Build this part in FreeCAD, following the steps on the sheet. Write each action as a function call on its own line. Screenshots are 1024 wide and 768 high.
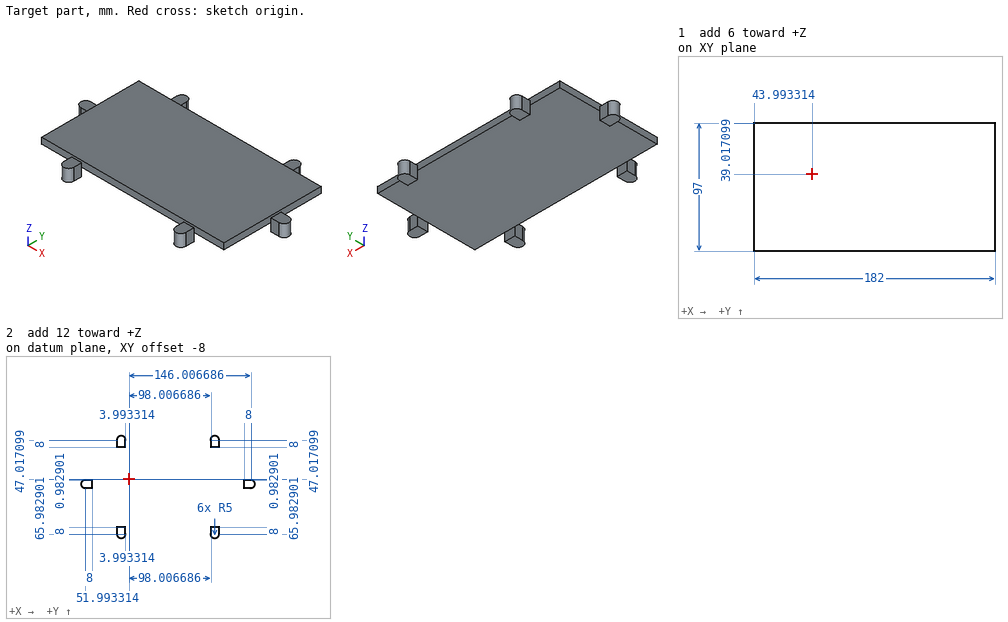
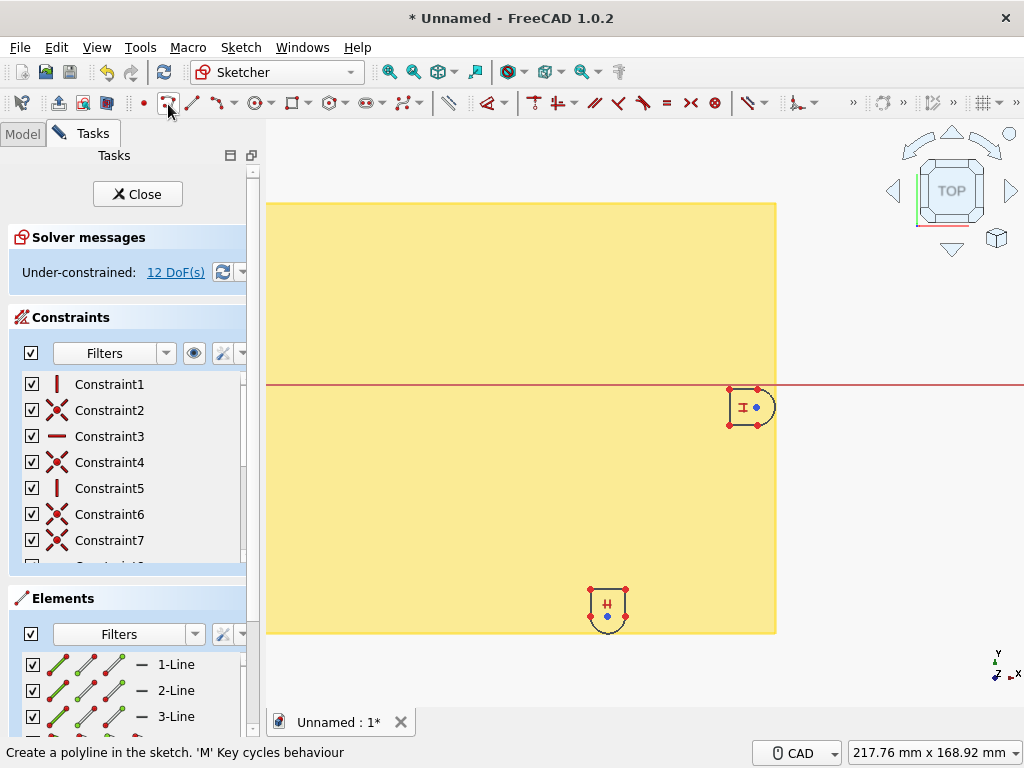
click(590, 222)
click(590, 250)
click(625, 250)
click(625, 222)
right_click(625, 222)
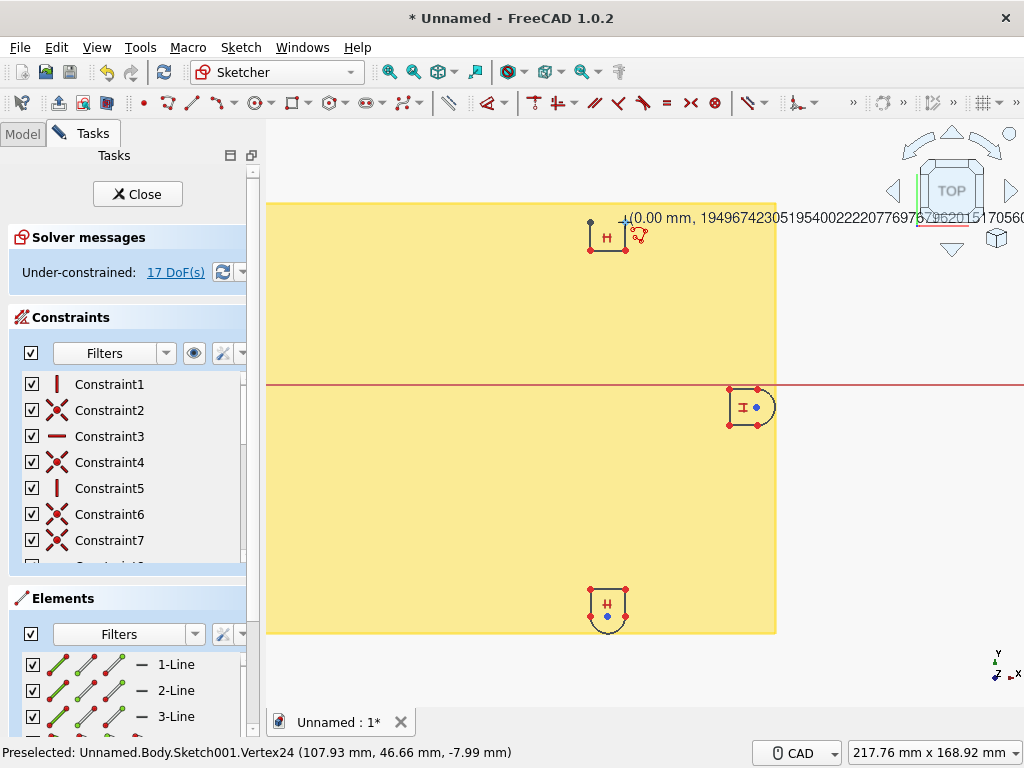
click(218, 104)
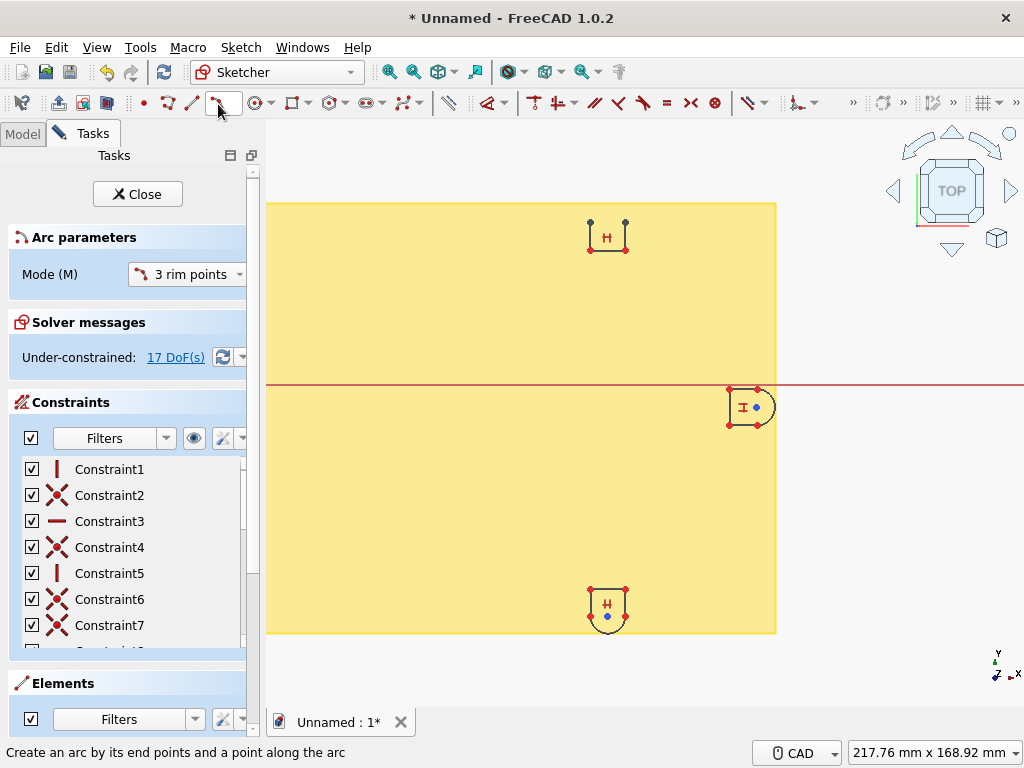
click(625, 223)
click(590, 223)
click(608, 204)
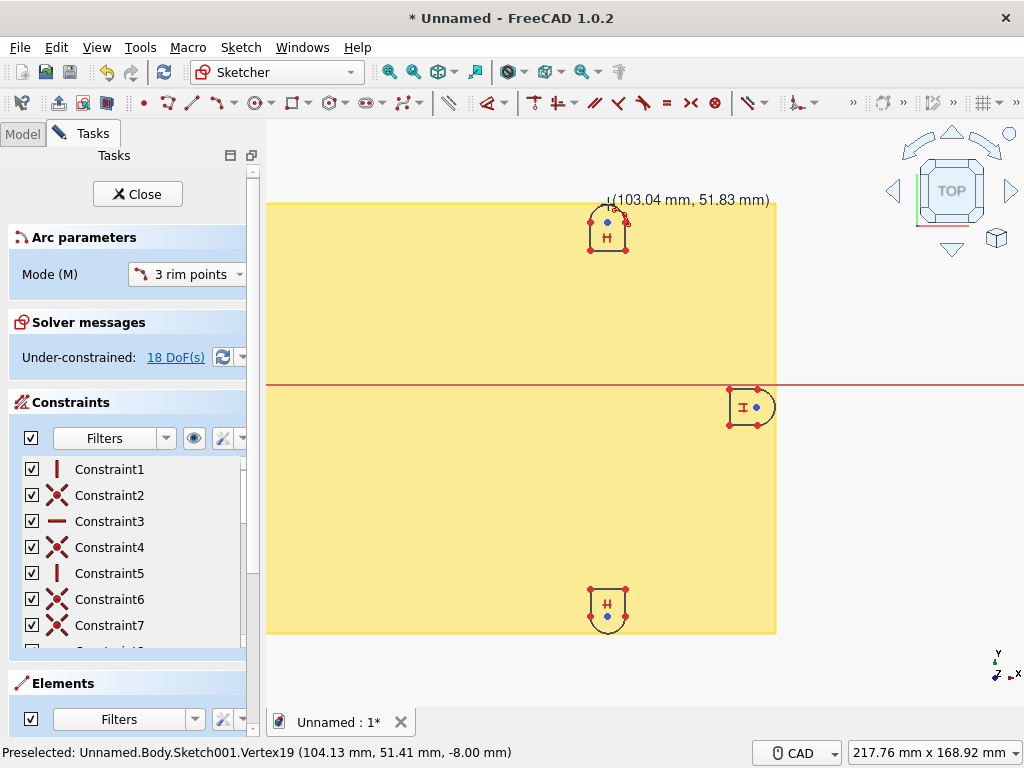
click(168, 104)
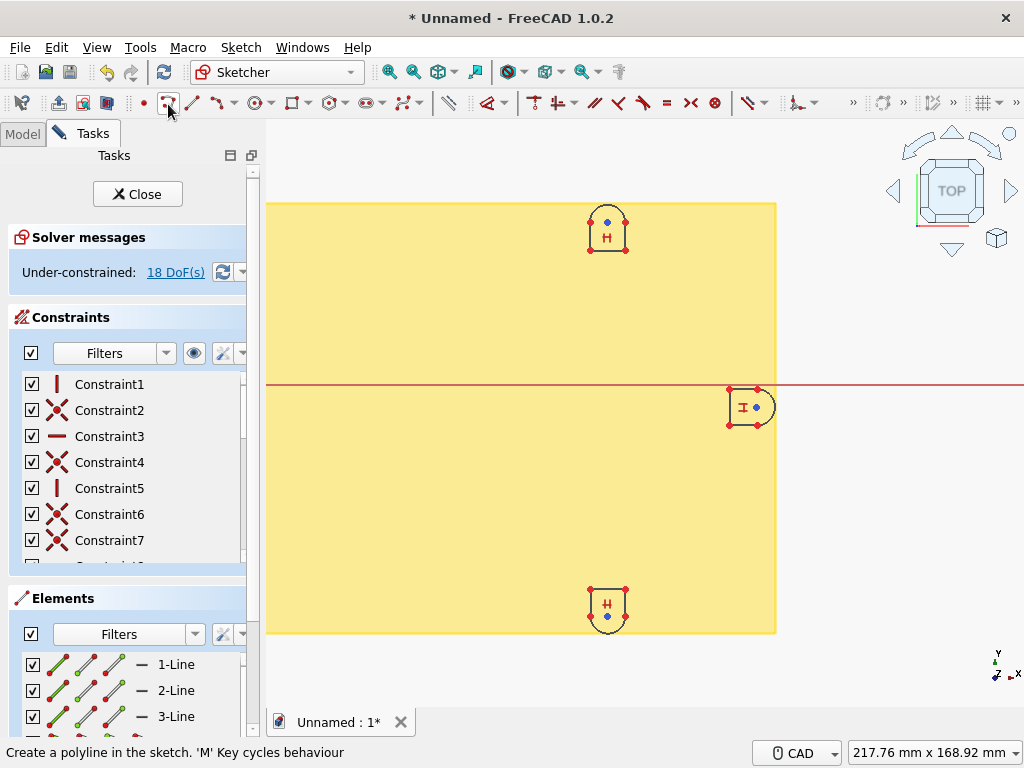
scroll(775, 406, down, 3)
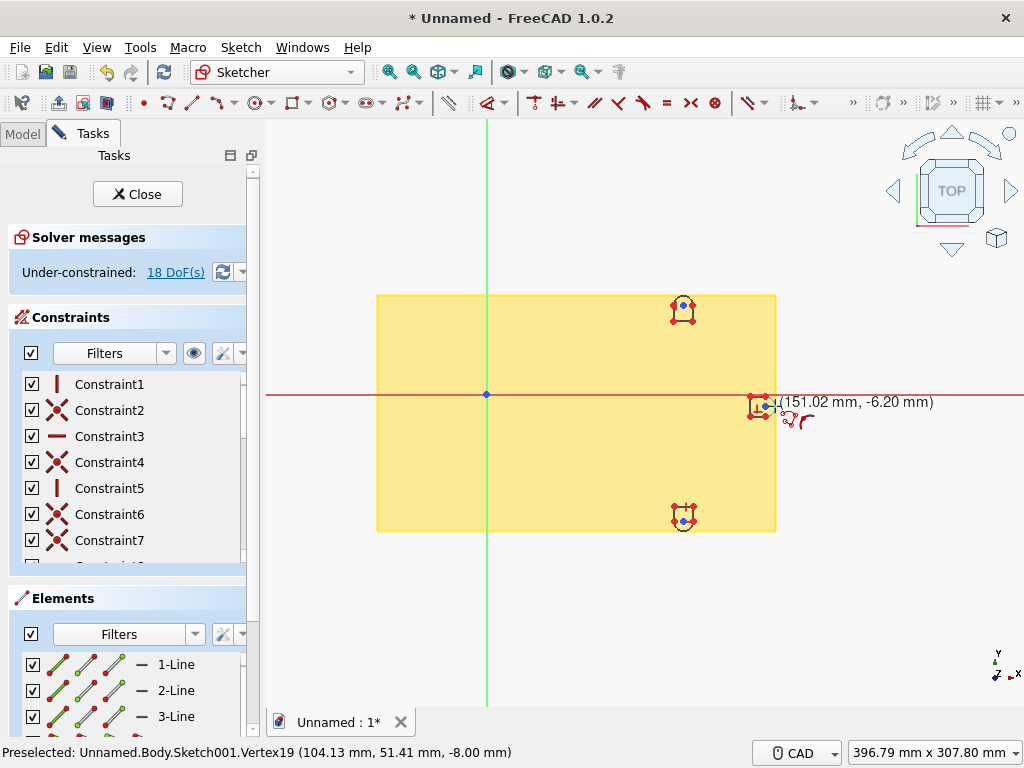
click(460, 305)
click(460, 320)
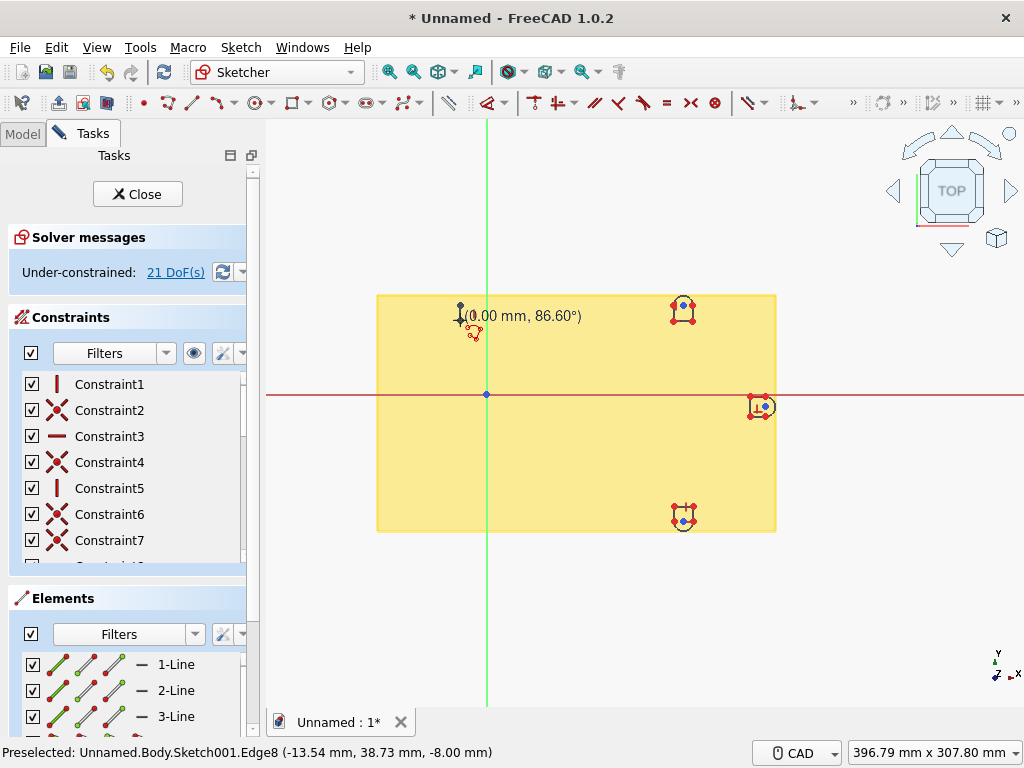
scroll(479, 320, up, 4)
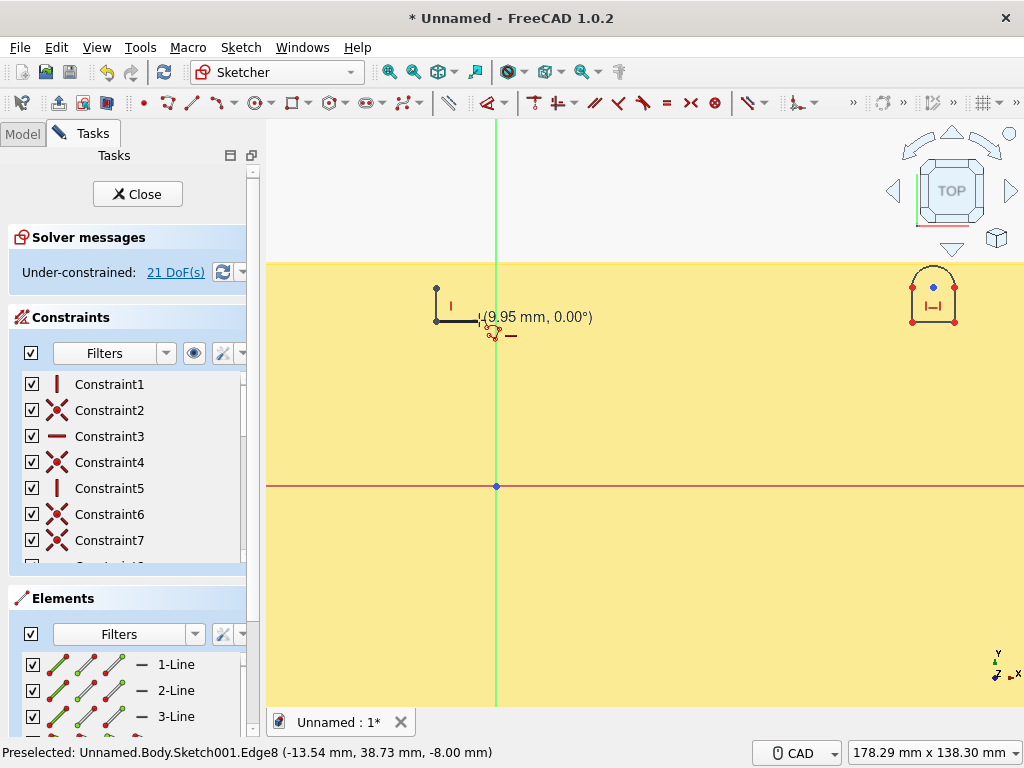
click(479, 320)
click(479, 286)
right_click(479, 286)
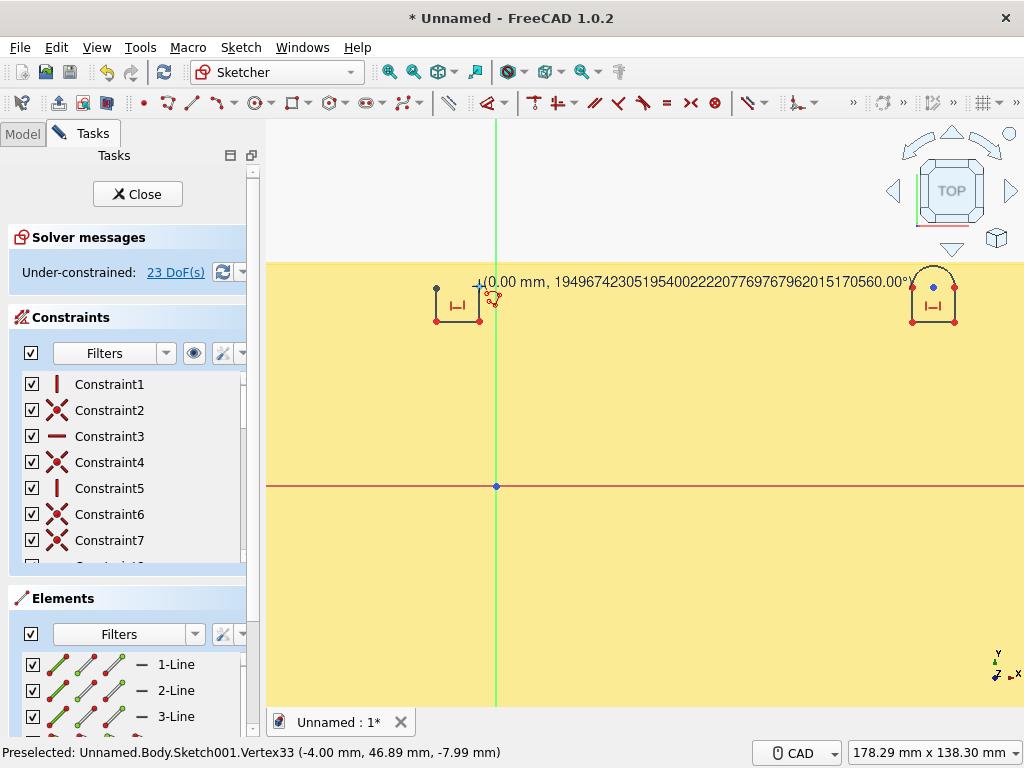
click(218, 104)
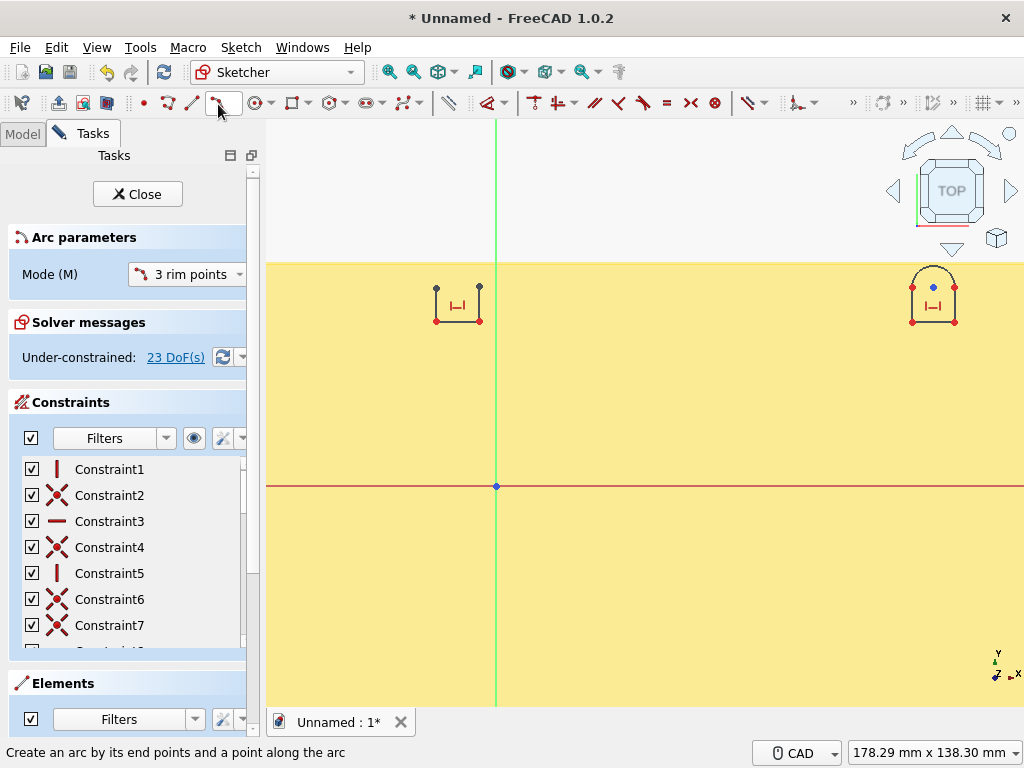
click(479, 287)
click(436, 288)
click(458, 265)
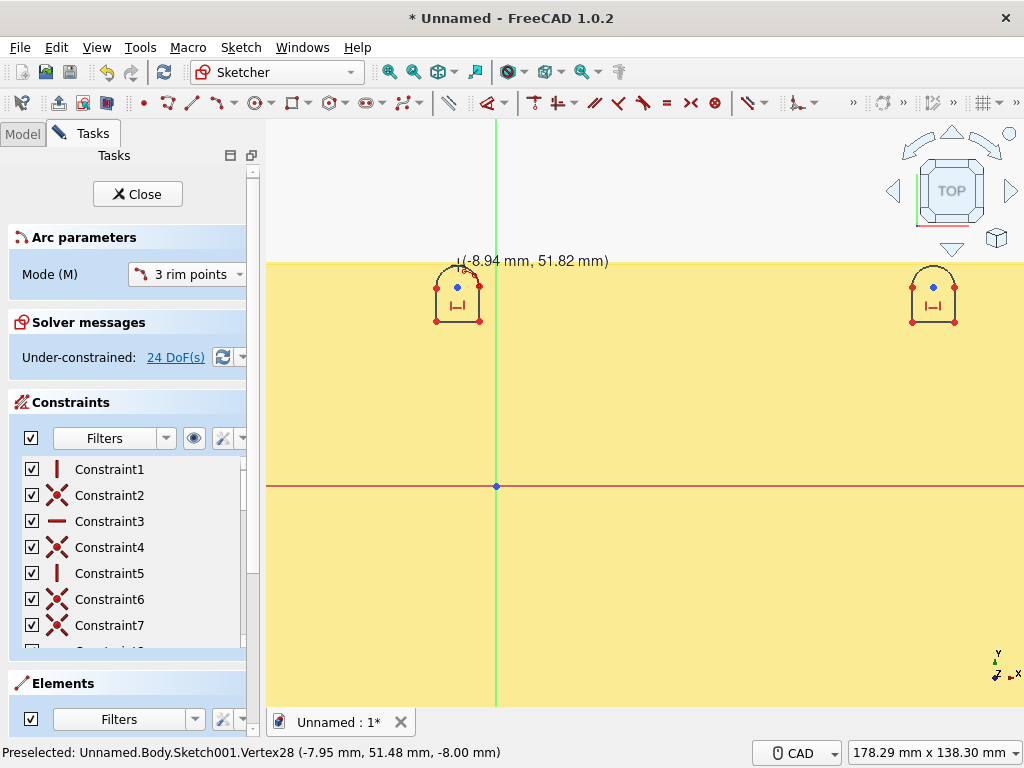
click(168, 104)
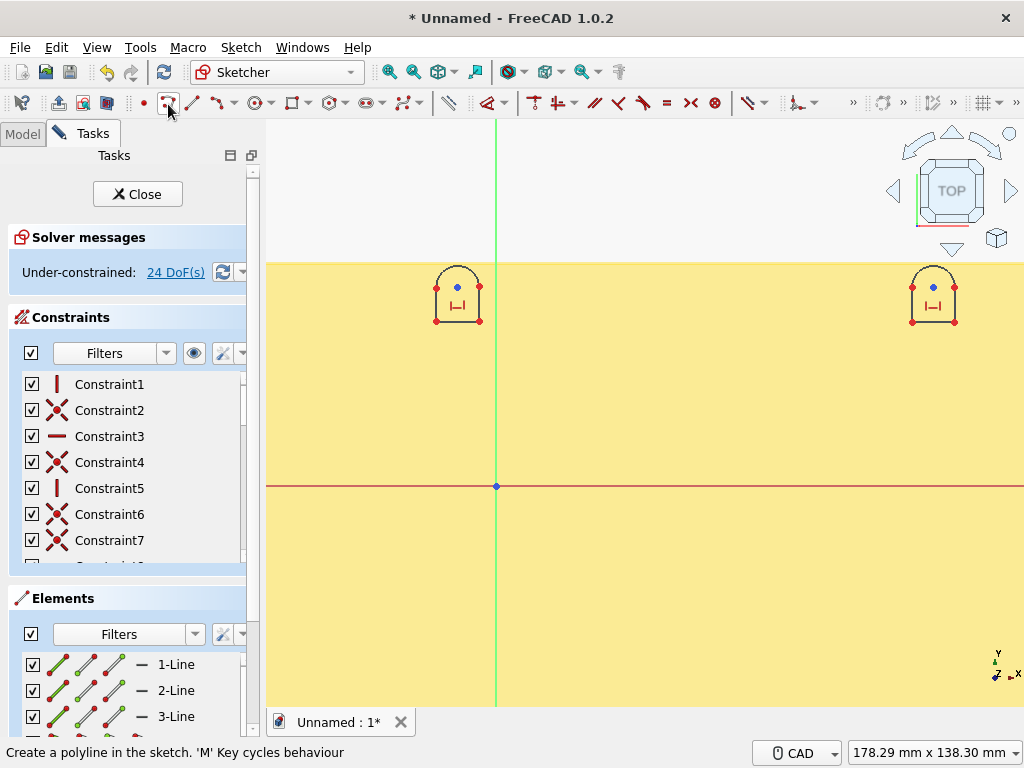
scroll(479, 320, down, 4)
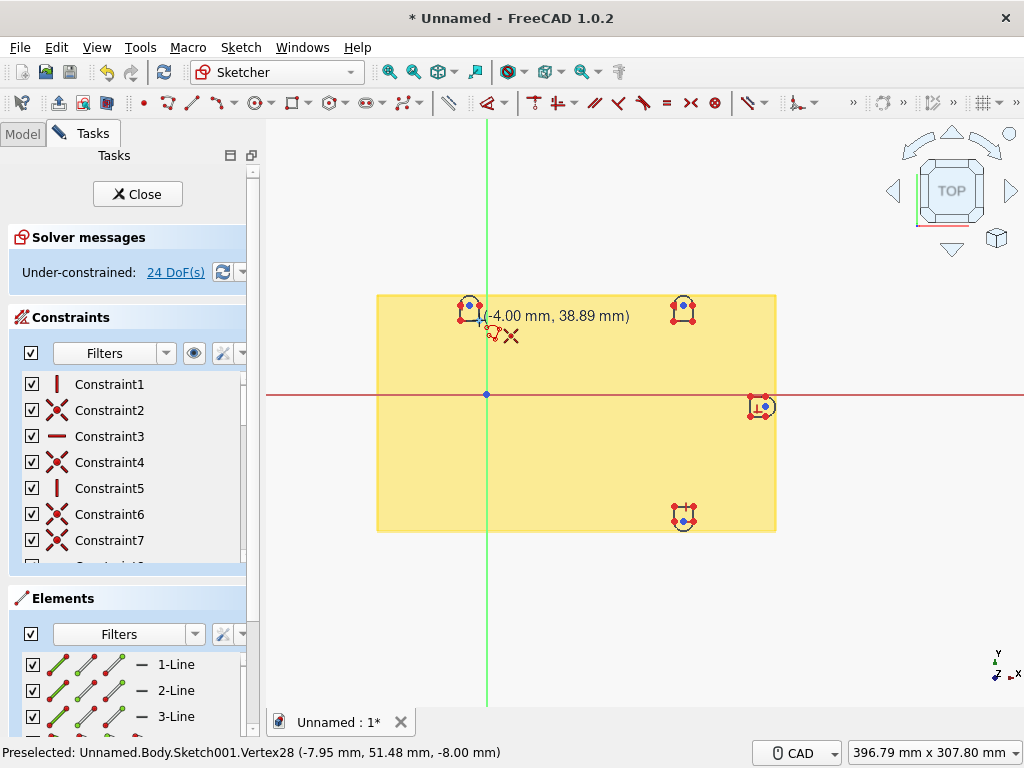
click(387, 416)
click(403, 416)